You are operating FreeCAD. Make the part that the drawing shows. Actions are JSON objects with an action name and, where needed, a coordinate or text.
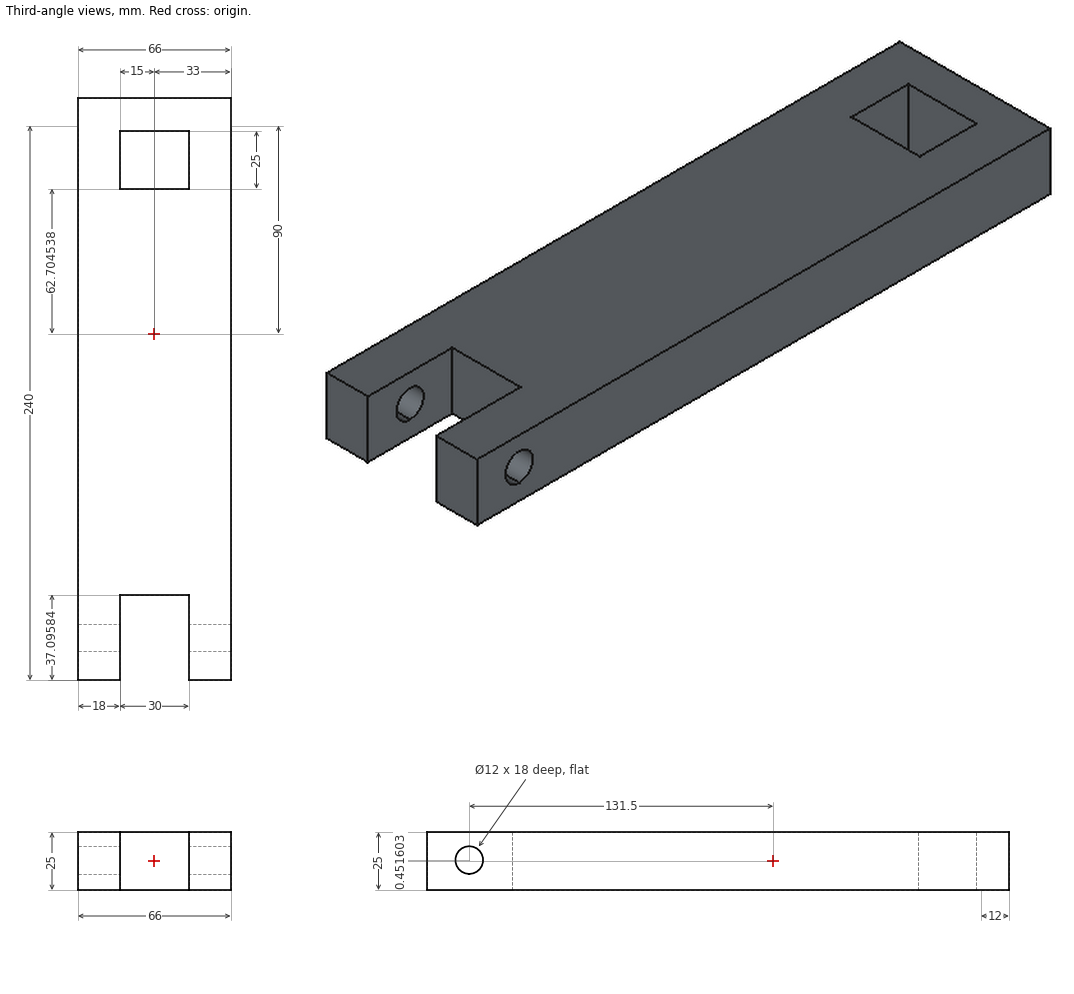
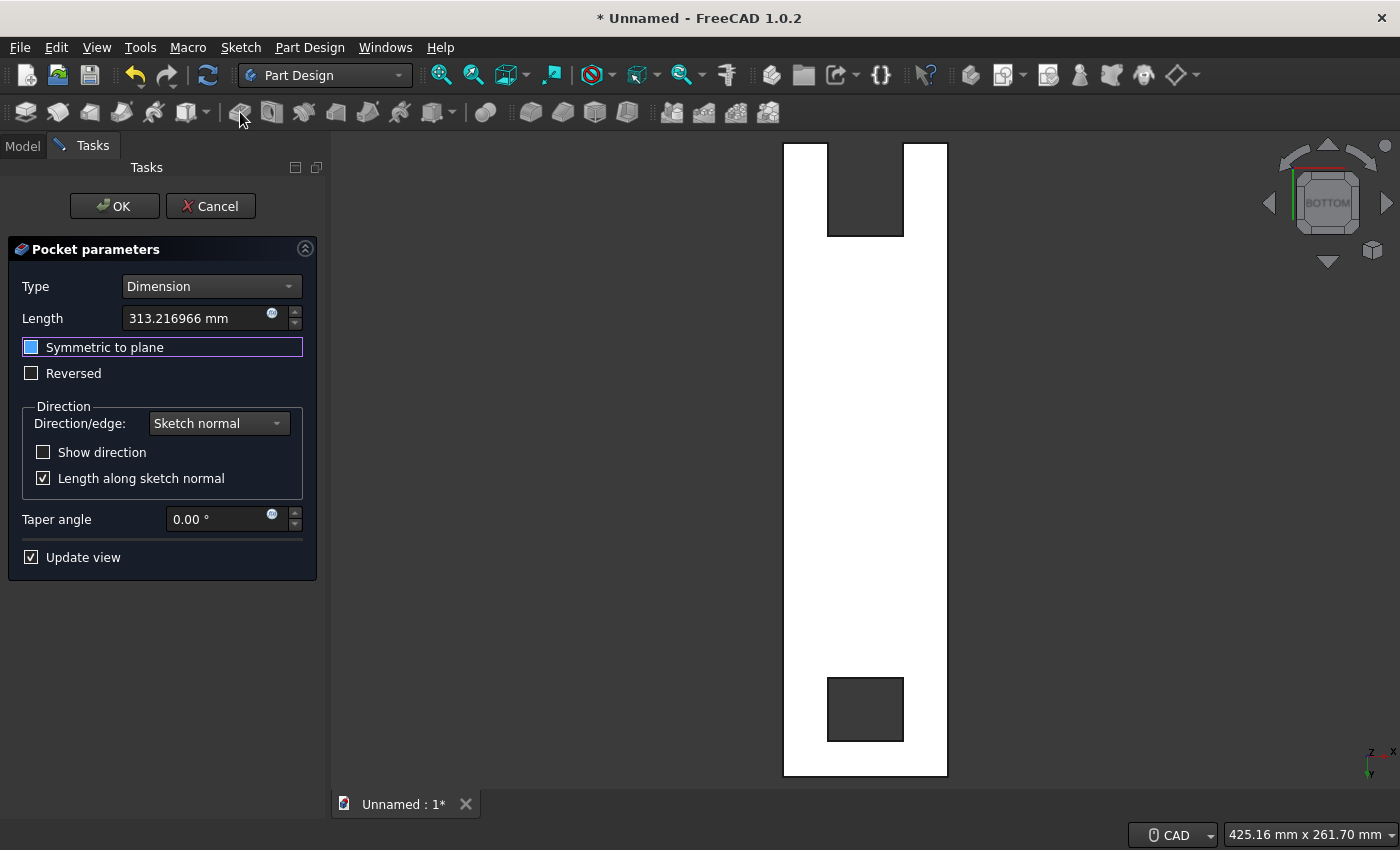
{"action": "left_click", "coordinate": [30, 347]}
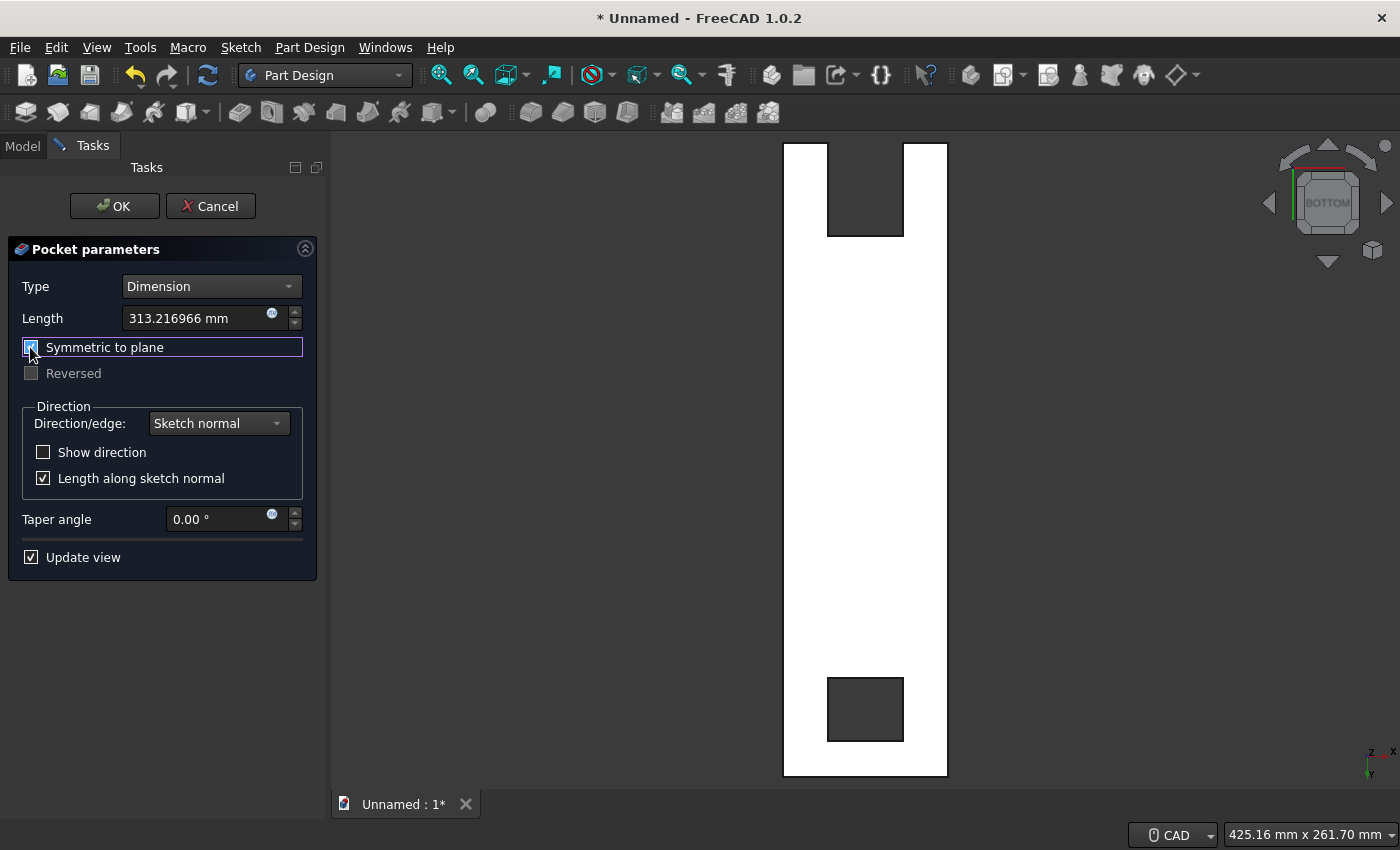
{"action": "left_click", "coordinate": [115, 206]}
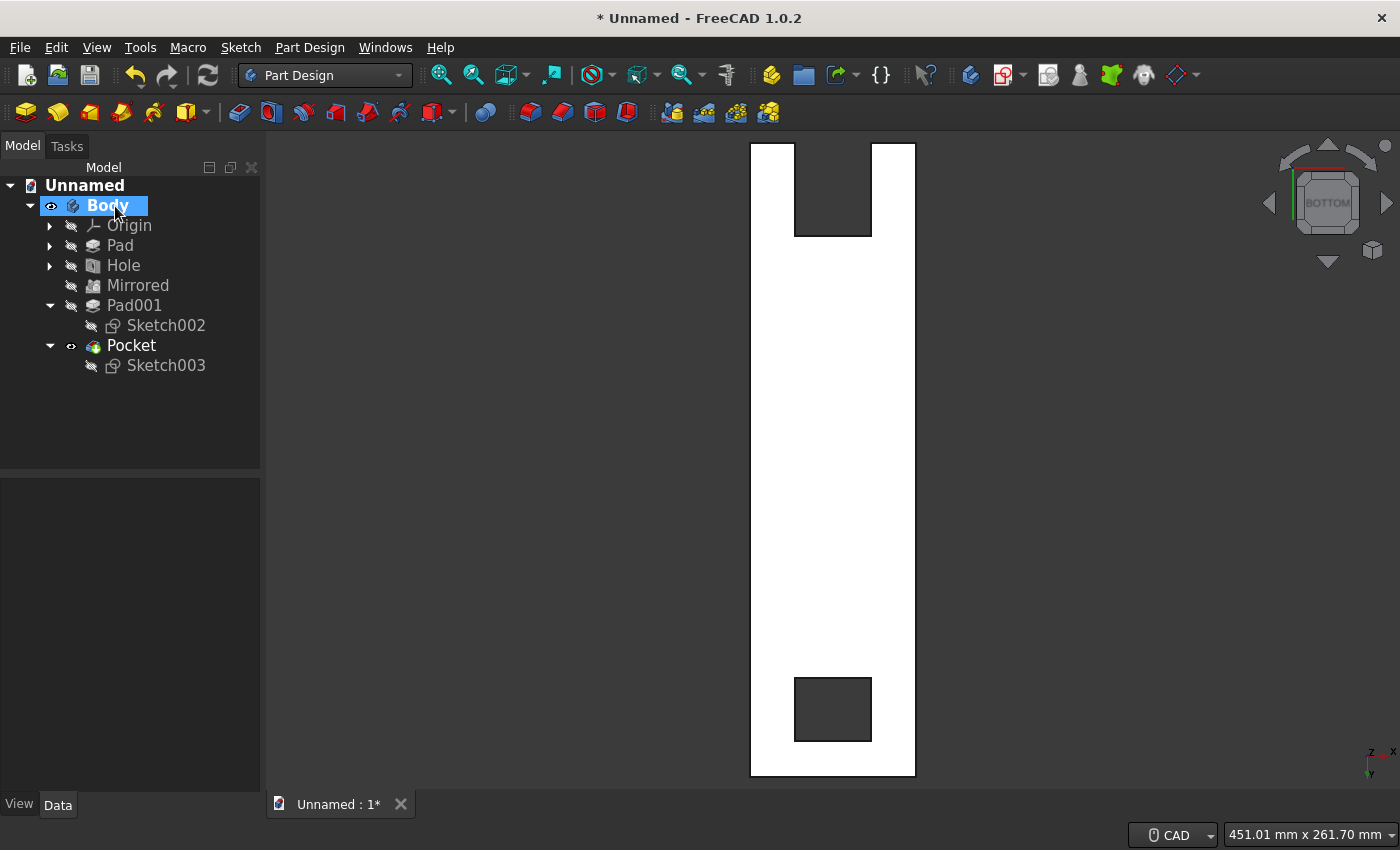
{"action": "key", "text": "0"}